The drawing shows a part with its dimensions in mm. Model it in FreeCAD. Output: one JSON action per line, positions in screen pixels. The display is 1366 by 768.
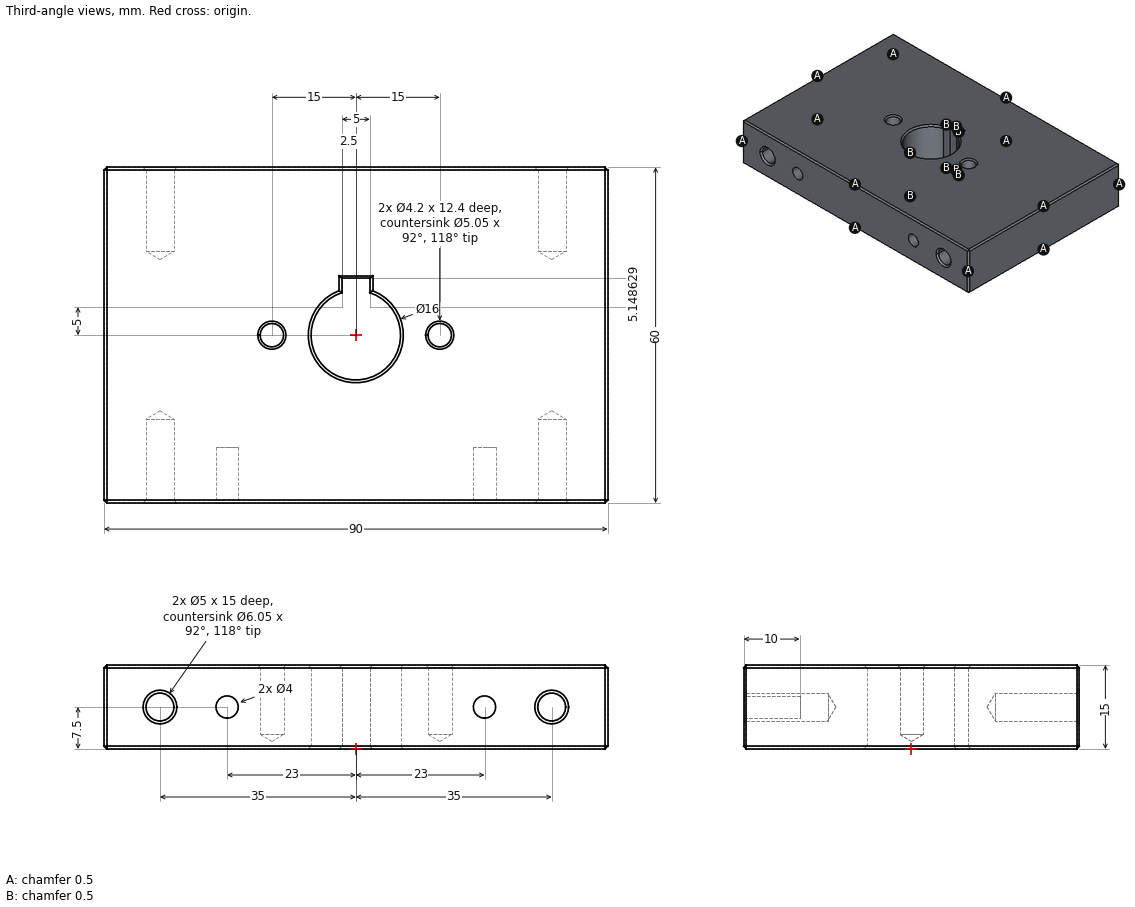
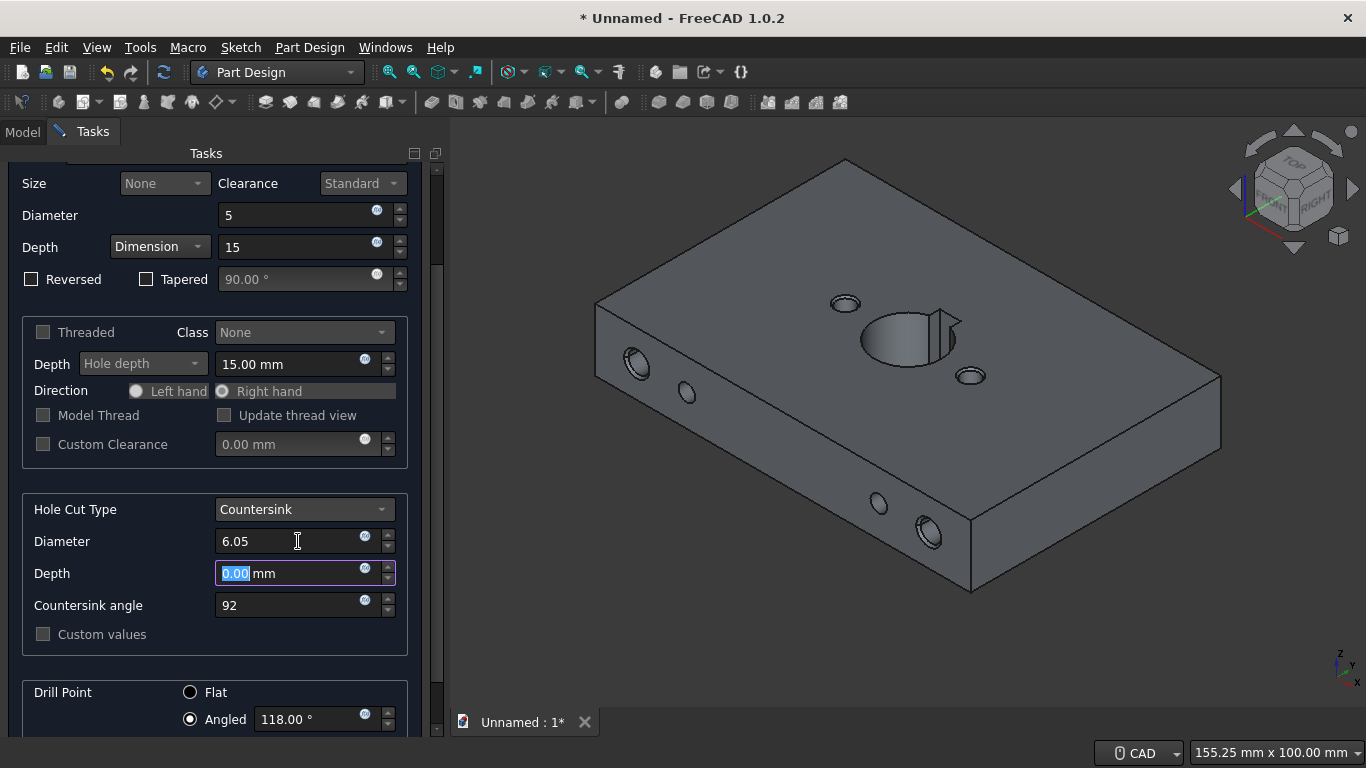
{"action": "scroll", "coordinate": [437, 450], "scroll_direction": "up", "scroll_amount": 3}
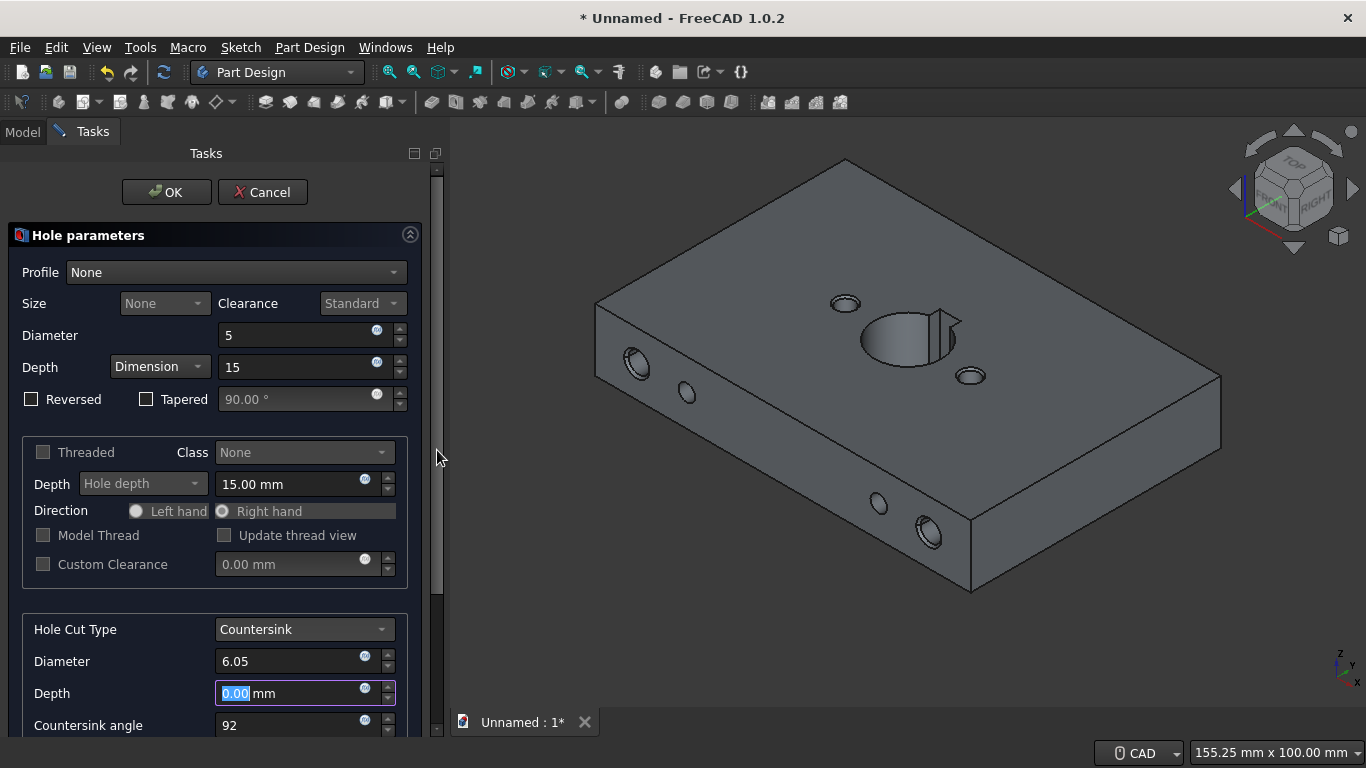
{"action": "left_click", "coordinate": [167, 192]}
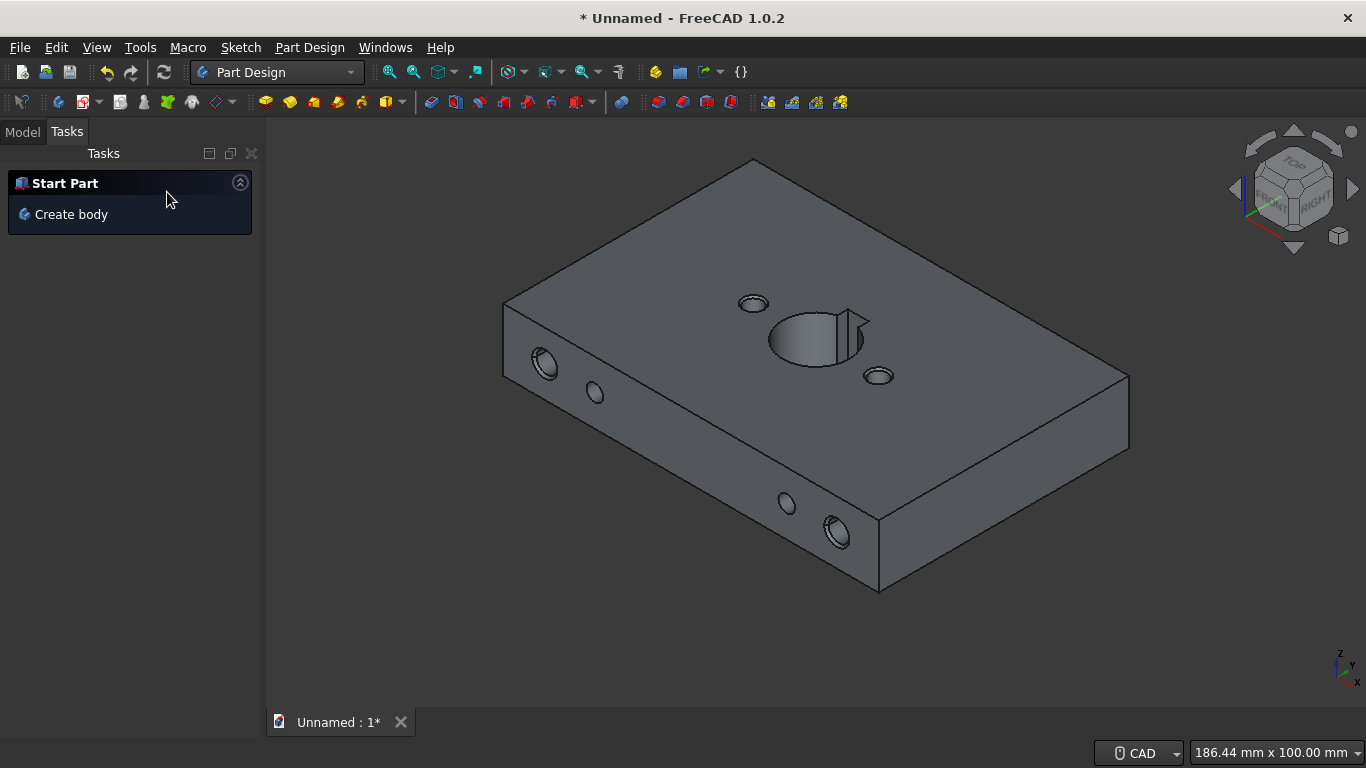
{"action": "left_click", "coordinate": [1075, 442]}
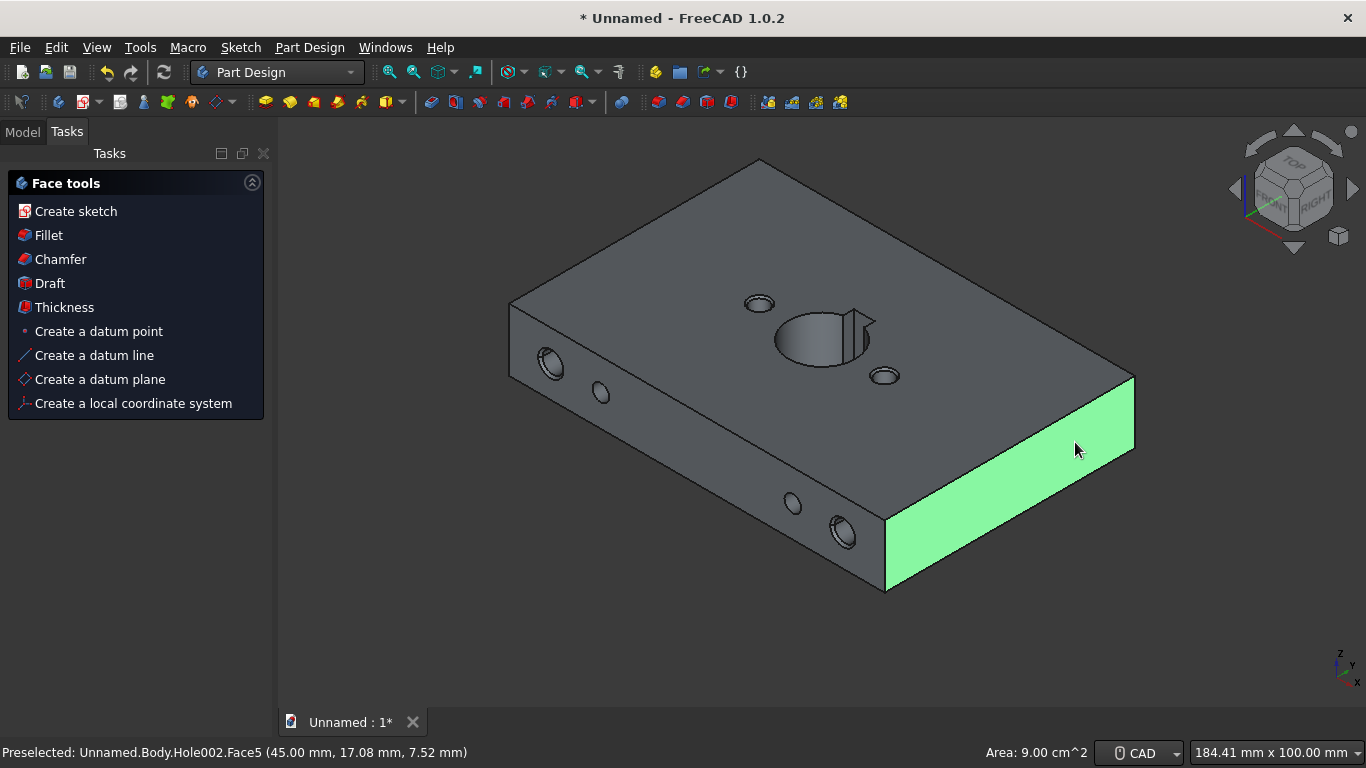
{"action": "left_click", "coordinate": [697, 411], "text": "ctrl"}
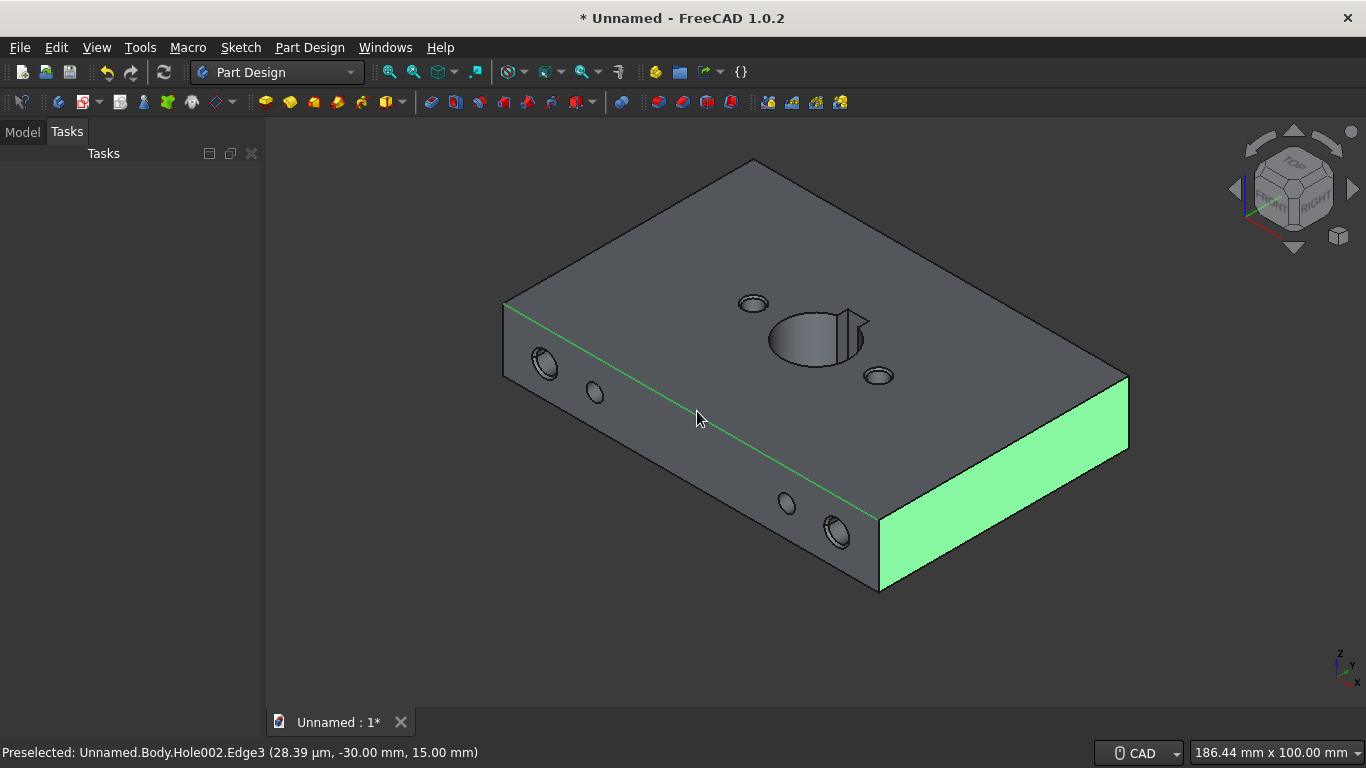
{"action": "key", "text": "2"}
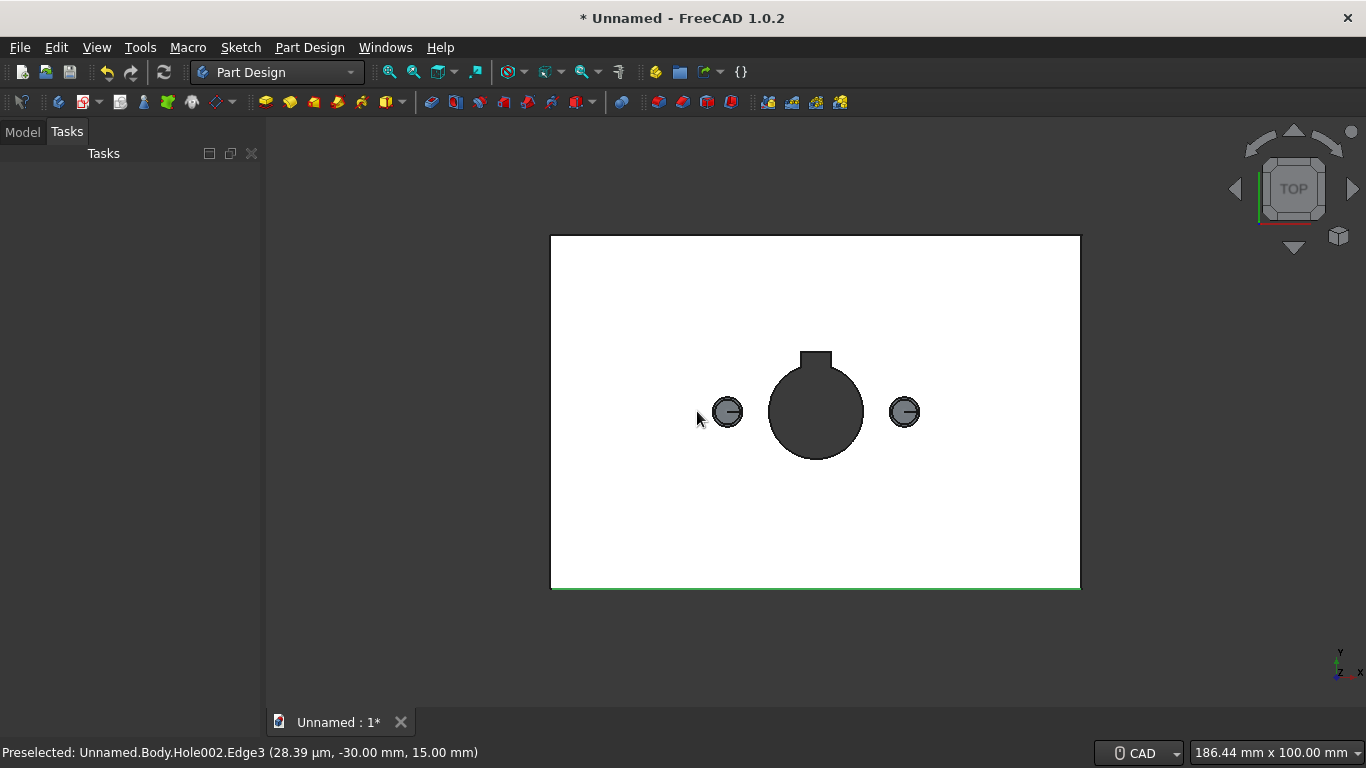
{"action": "left_click", "coordinate": [816, 234], "text": "ctrl"}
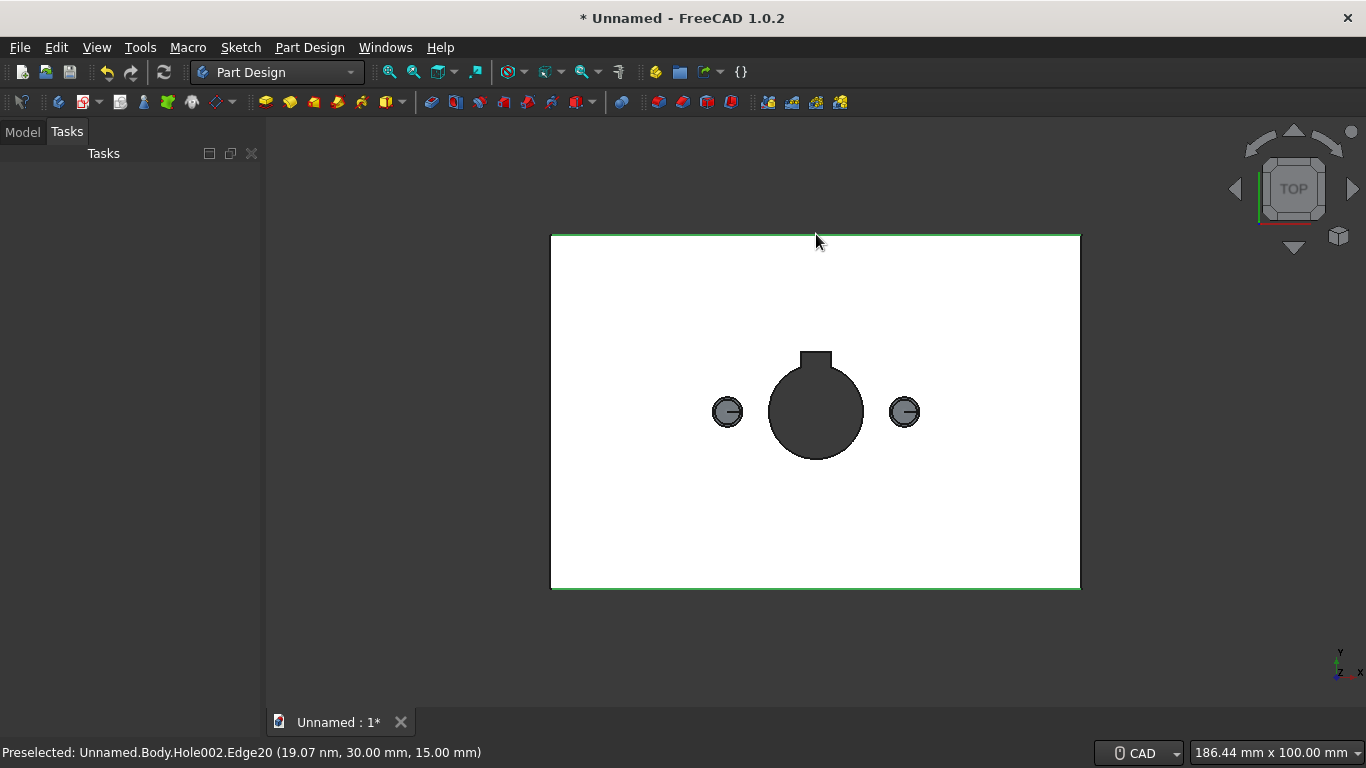
{"action": "key", "text": "0"}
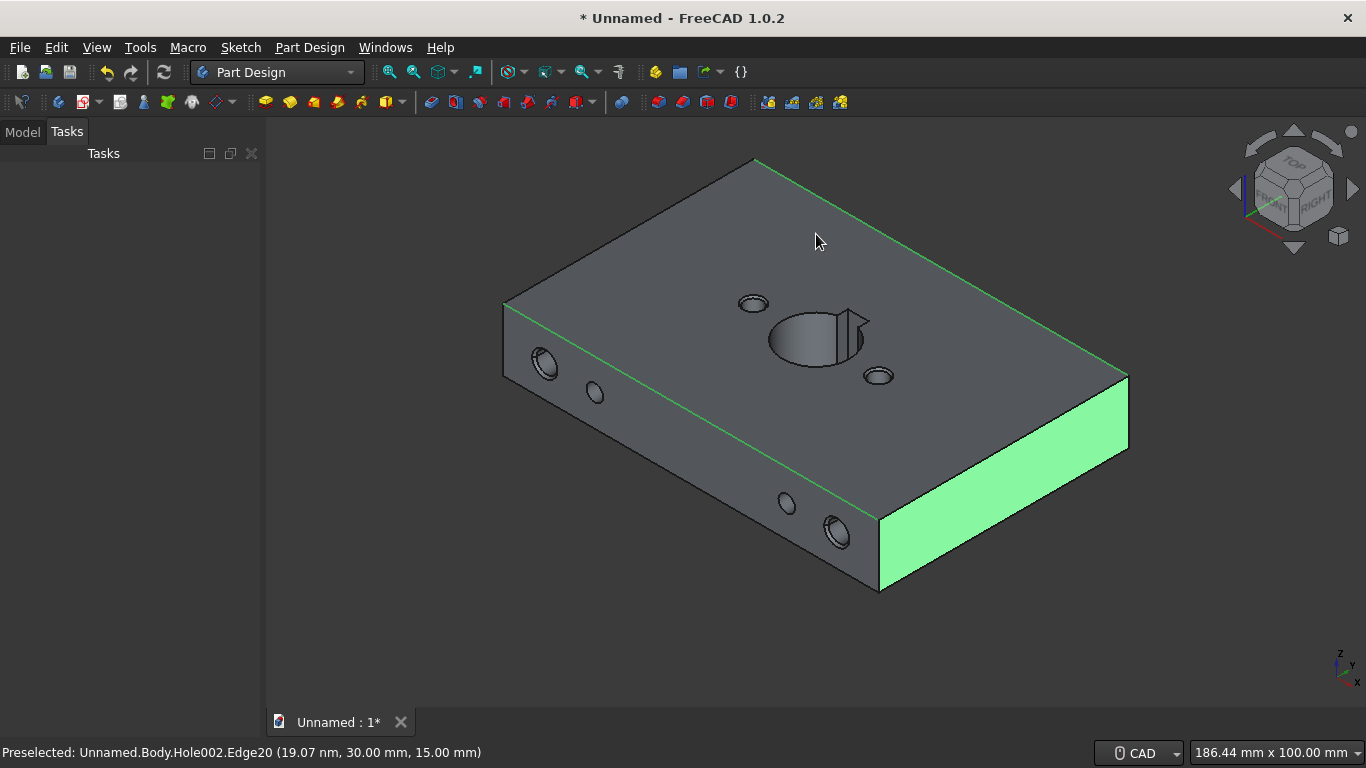
{"action": "key", "text": "1"}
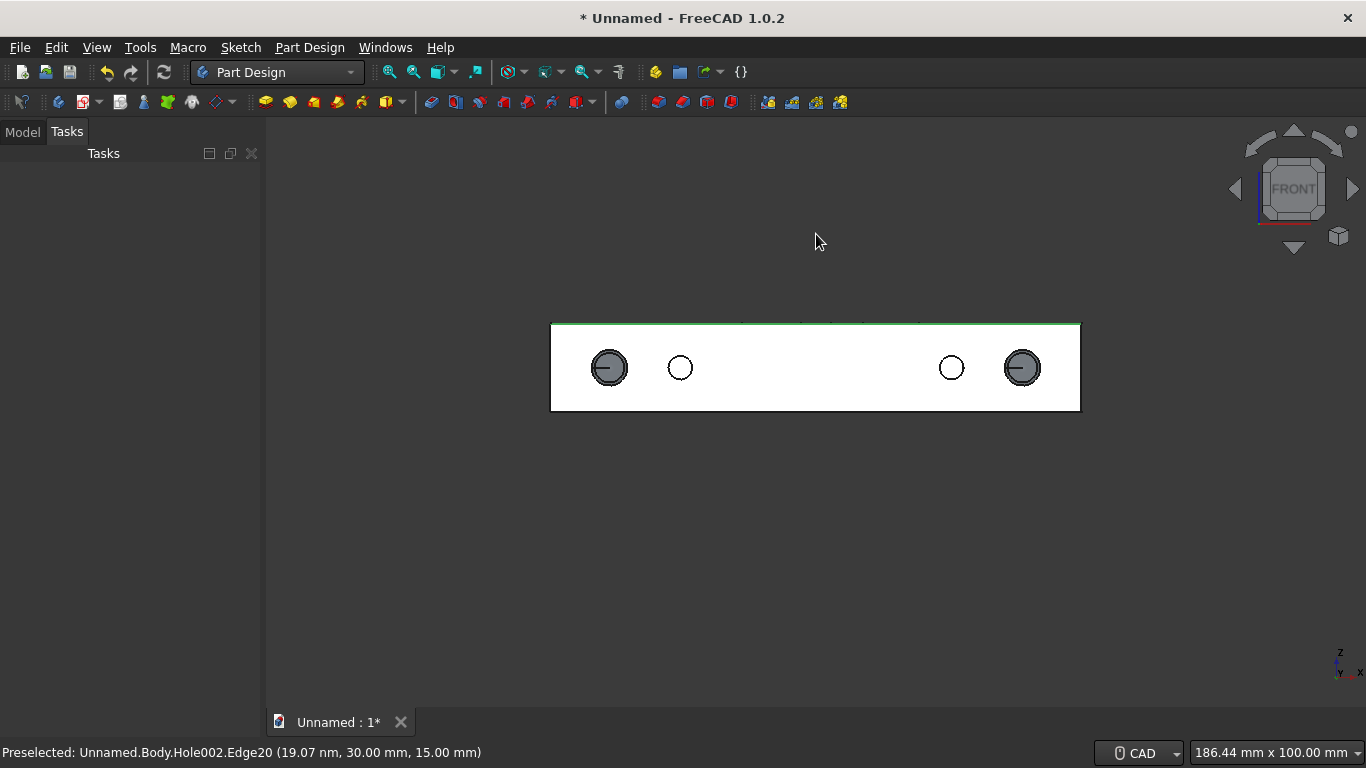
{"action": "left_click", "coordinate": [816, 411], "text": "ctrl"}